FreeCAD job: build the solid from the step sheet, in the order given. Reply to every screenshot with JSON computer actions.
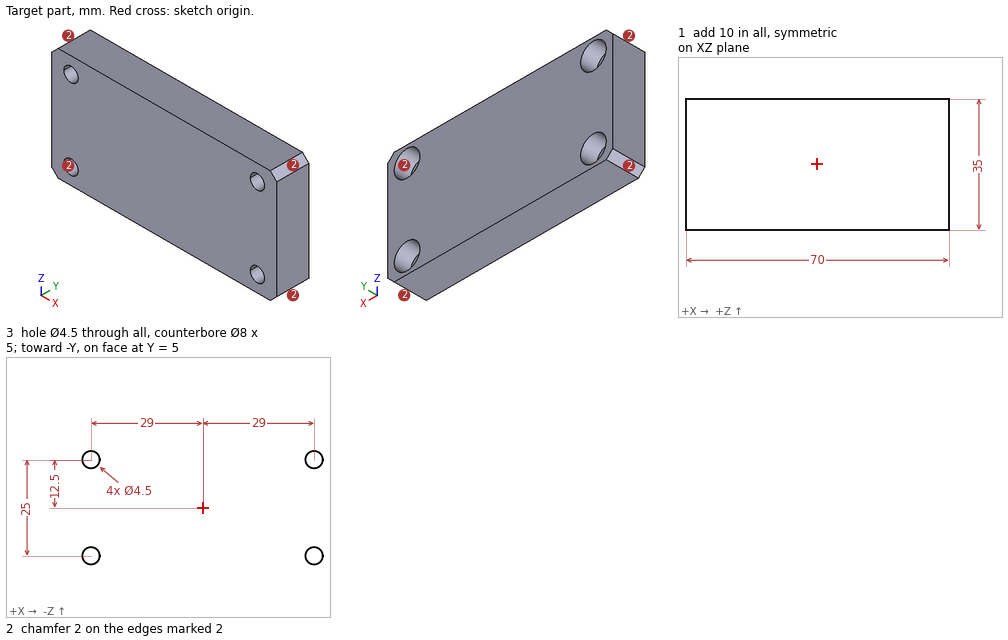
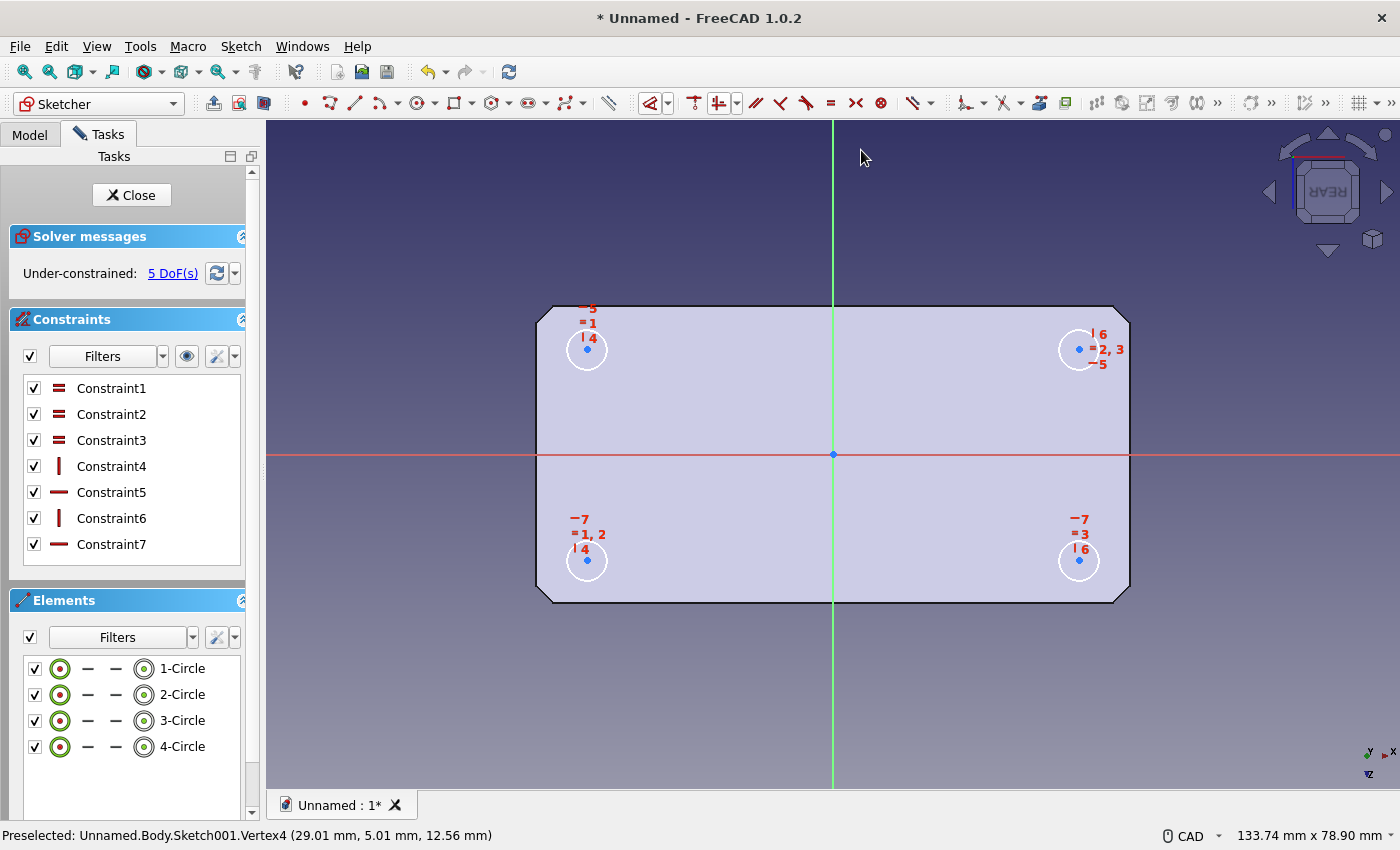
{"action": "left_click", "coordinate": [601, 336]}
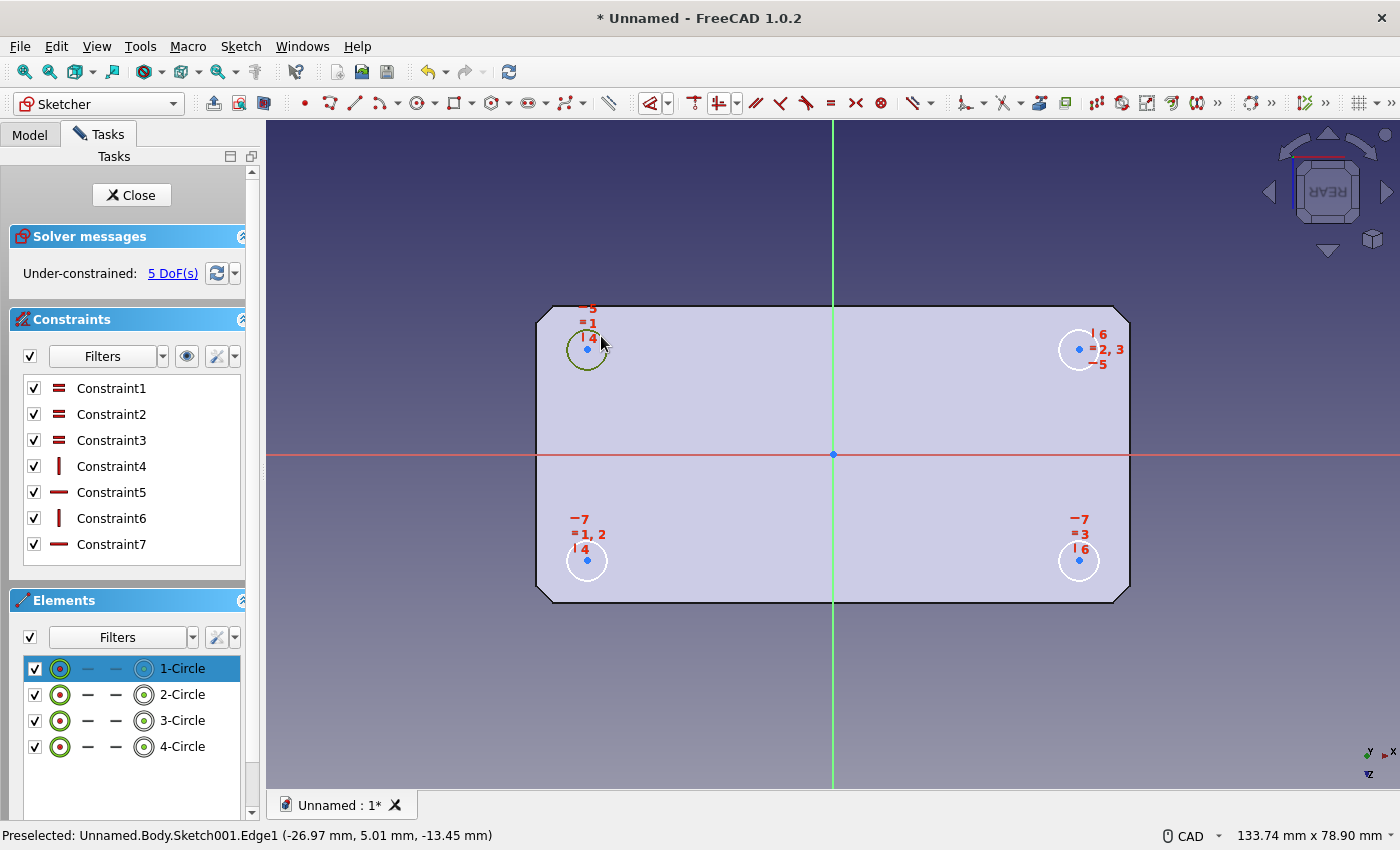
{"action": "left_click", "coordinate": [668, 104]}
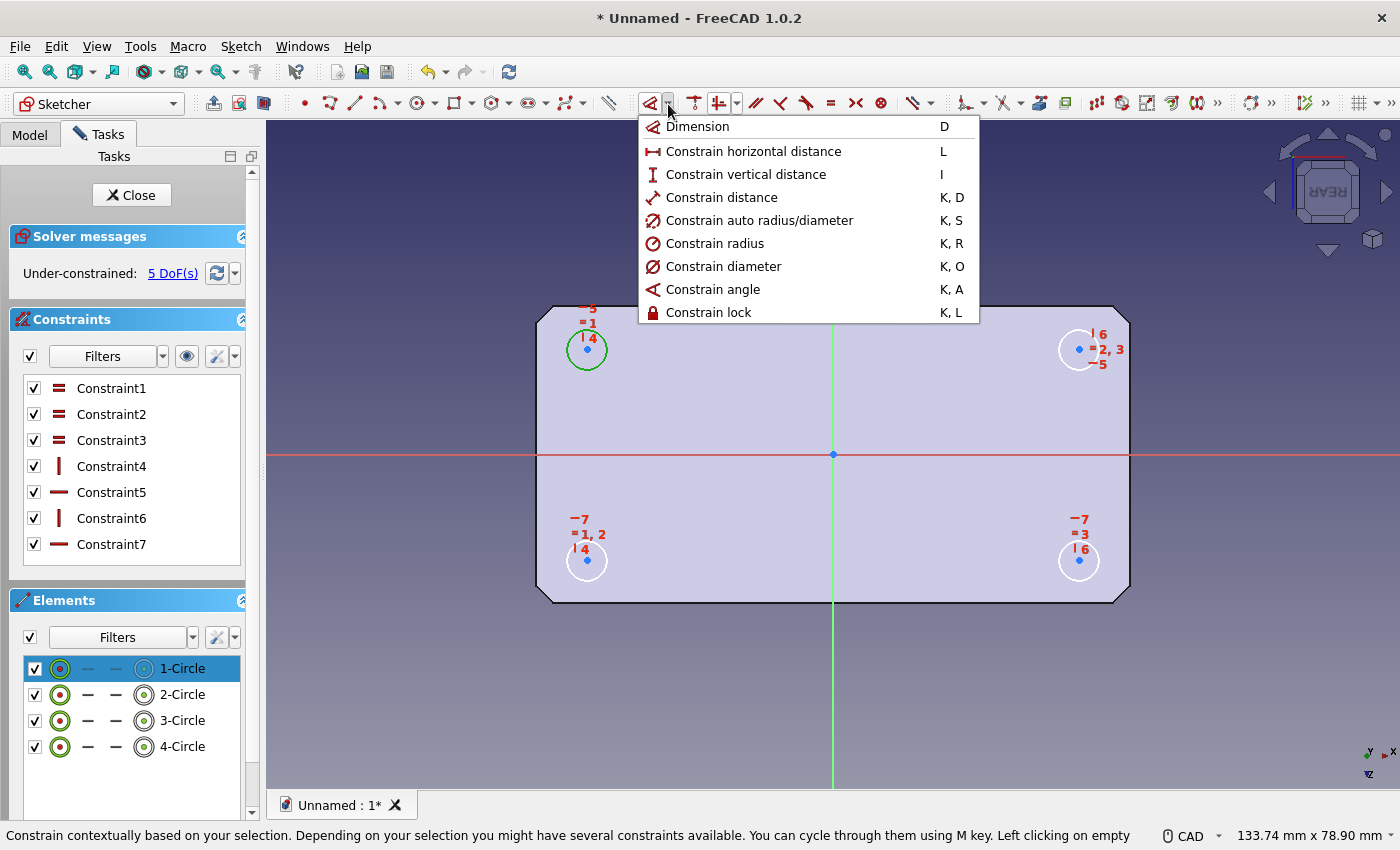
{"action": "left_click", "coordinate": [809, 266]}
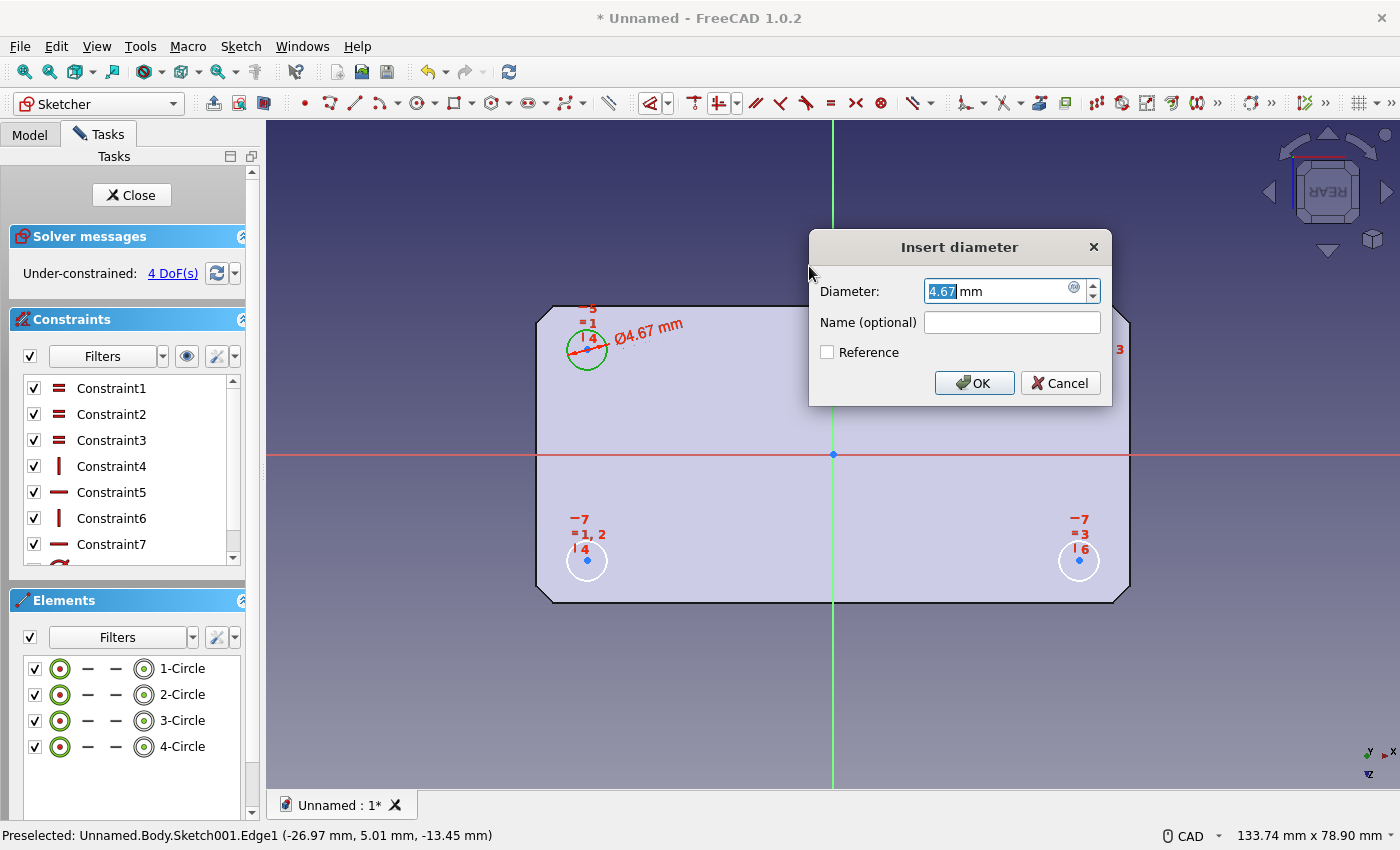
{"action": "type", "text": "4.5"}
{"action": "key", "text": "Return"}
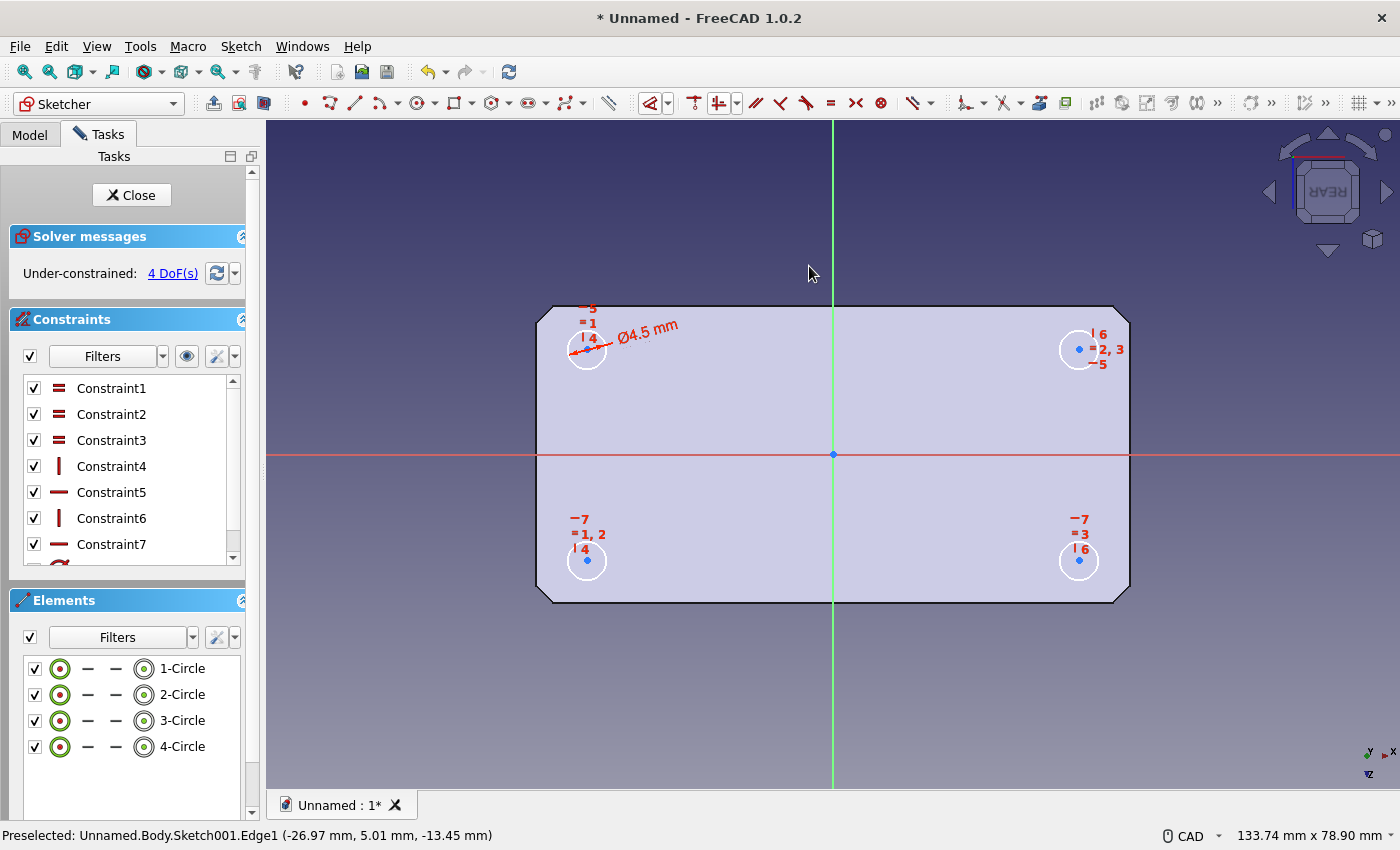
{"action": "left_click", "coordinate": [587, 350]}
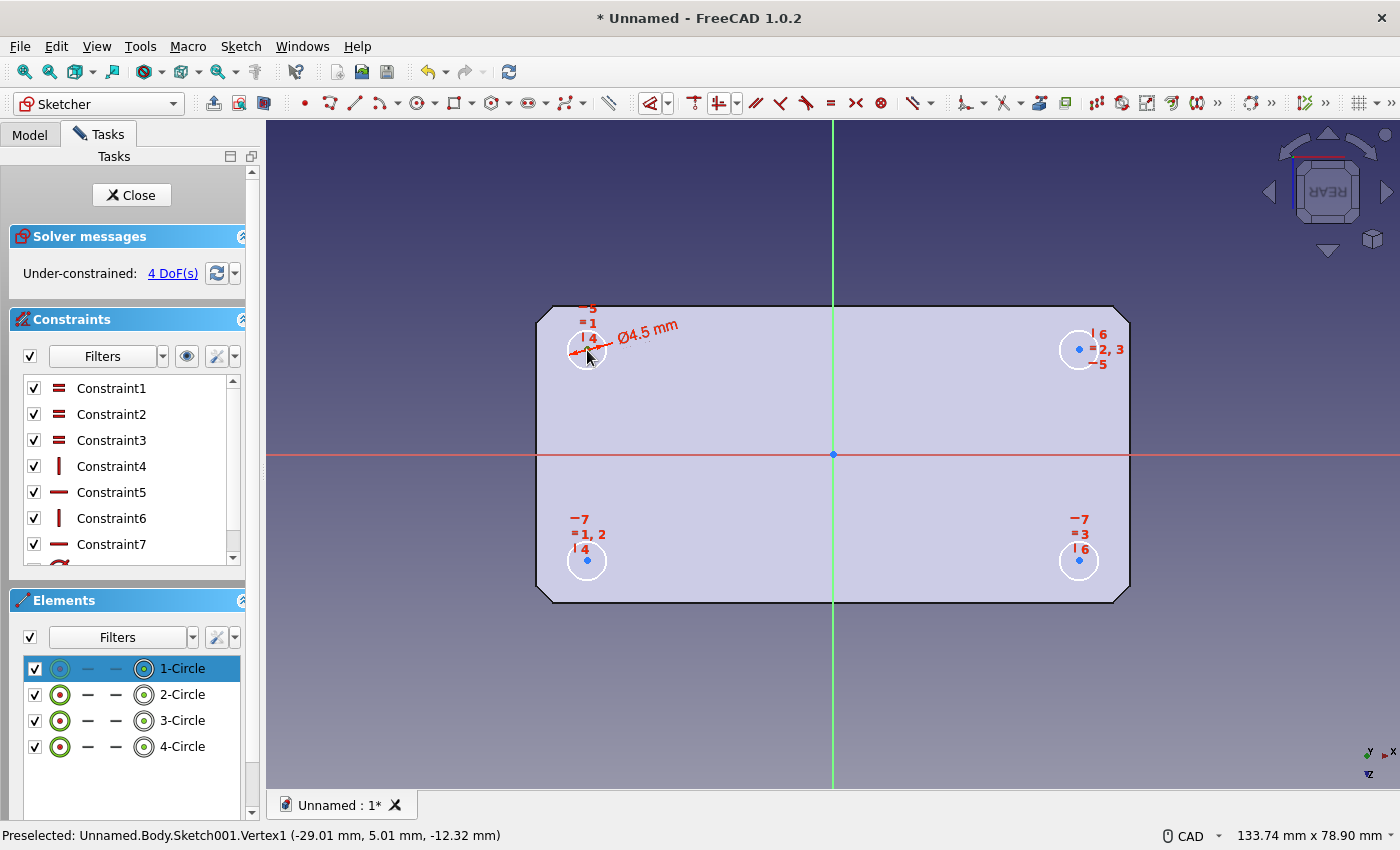
{"action": "key", "text": "l"}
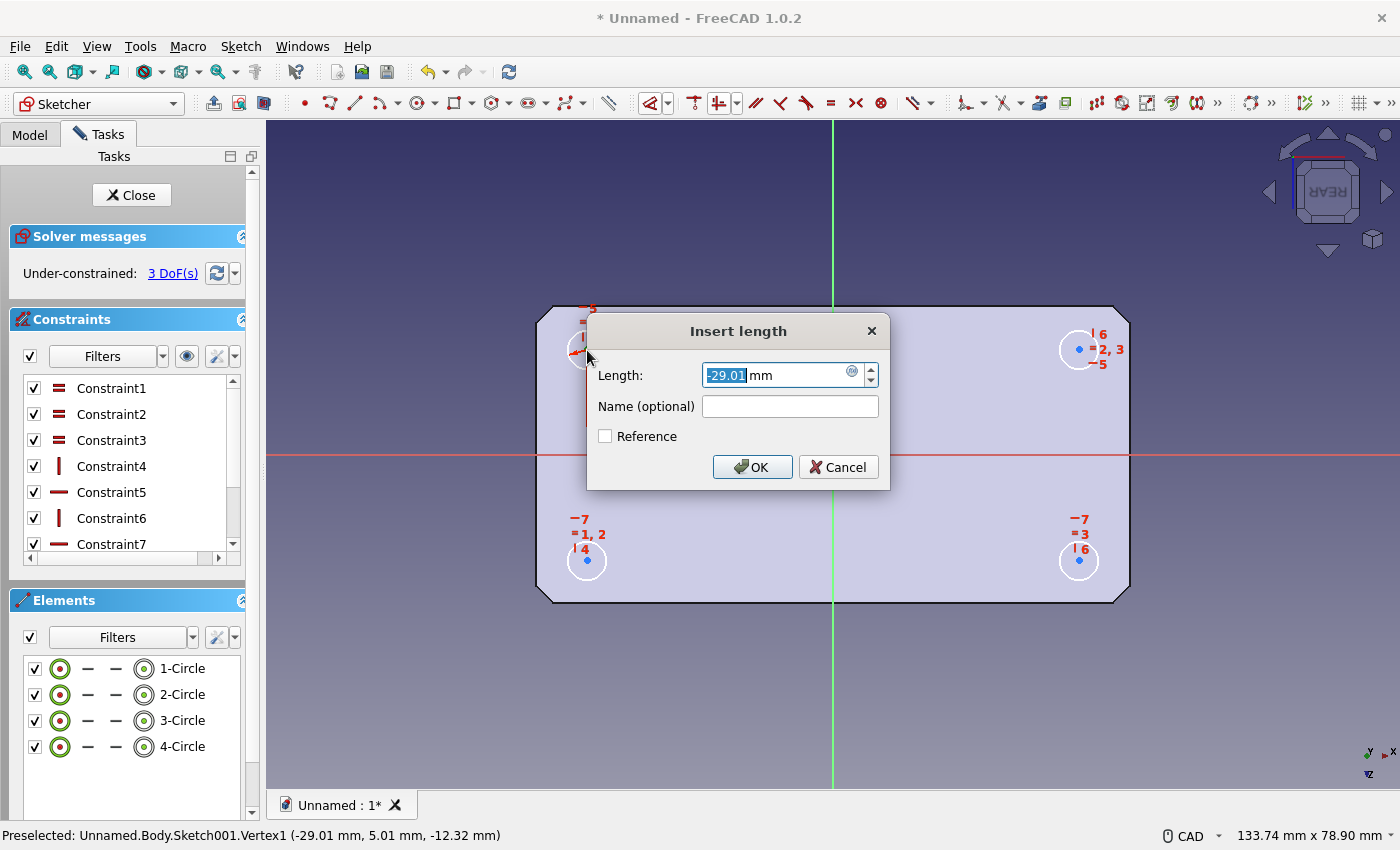
{"action": "type", "text": "-29"}
{"action": "key", "text": "Return"}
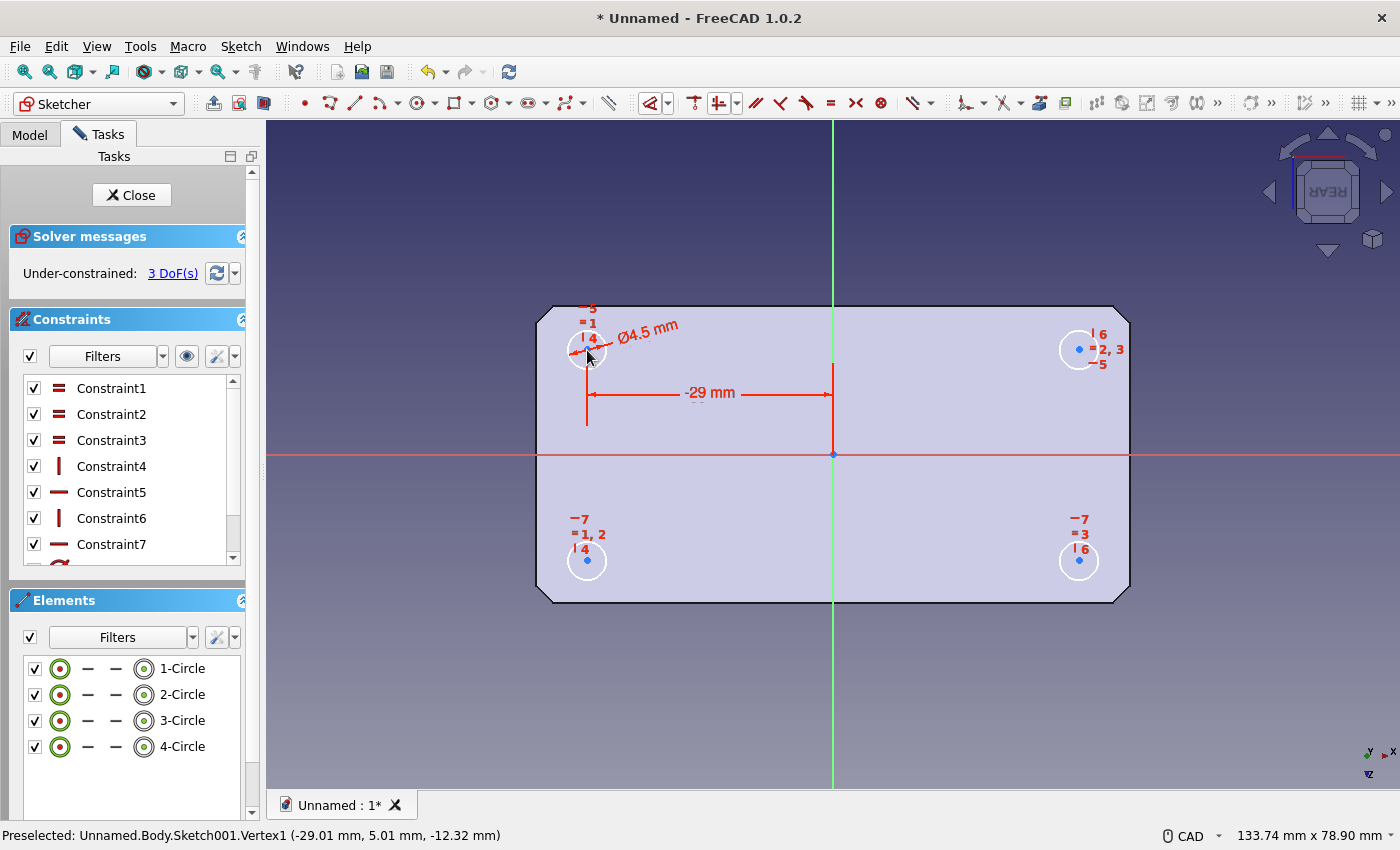
{"action": "left_click", "coordinate": [1079, 350]}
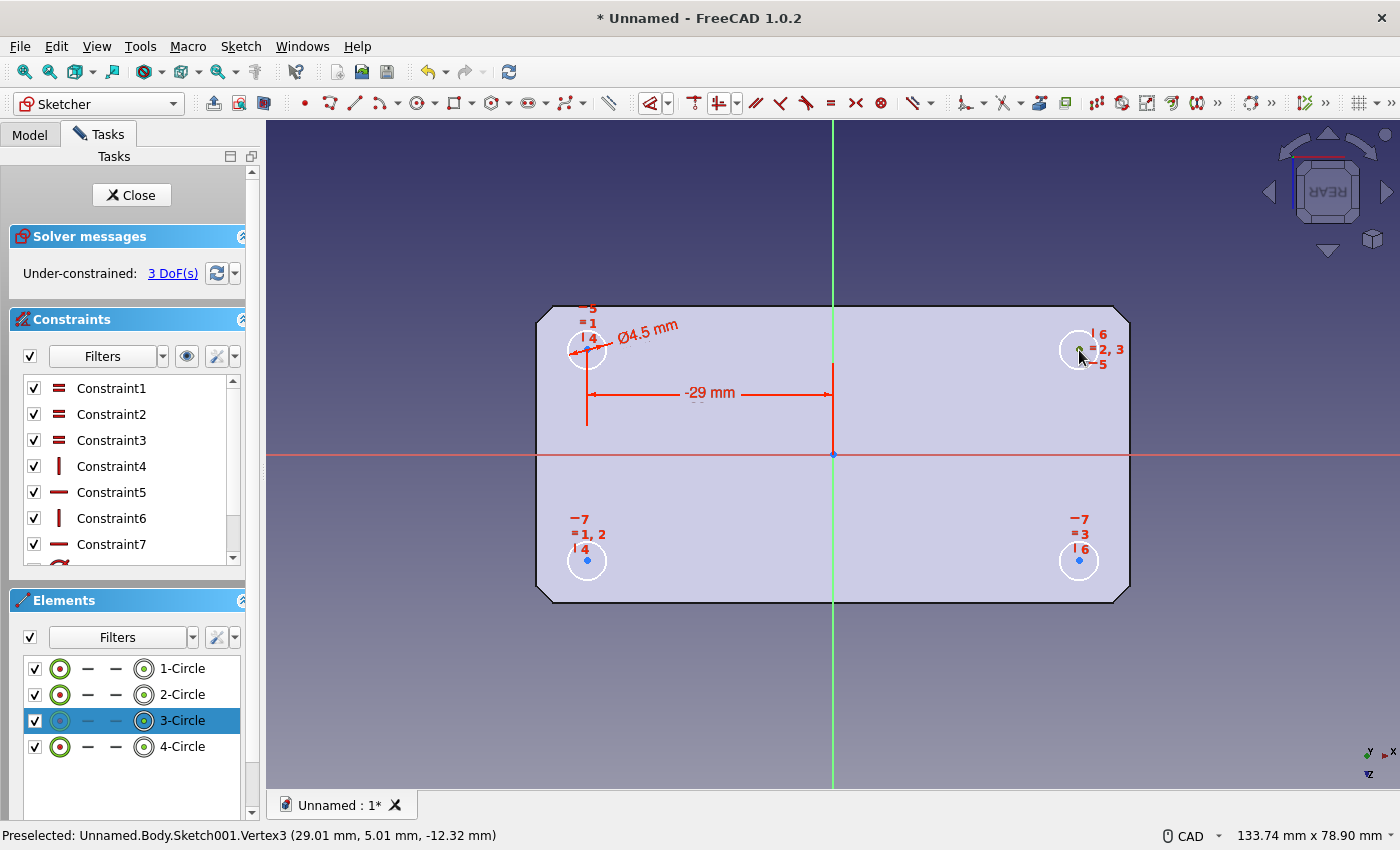
{"action": "left_click", "coordinate": [668, 104]}